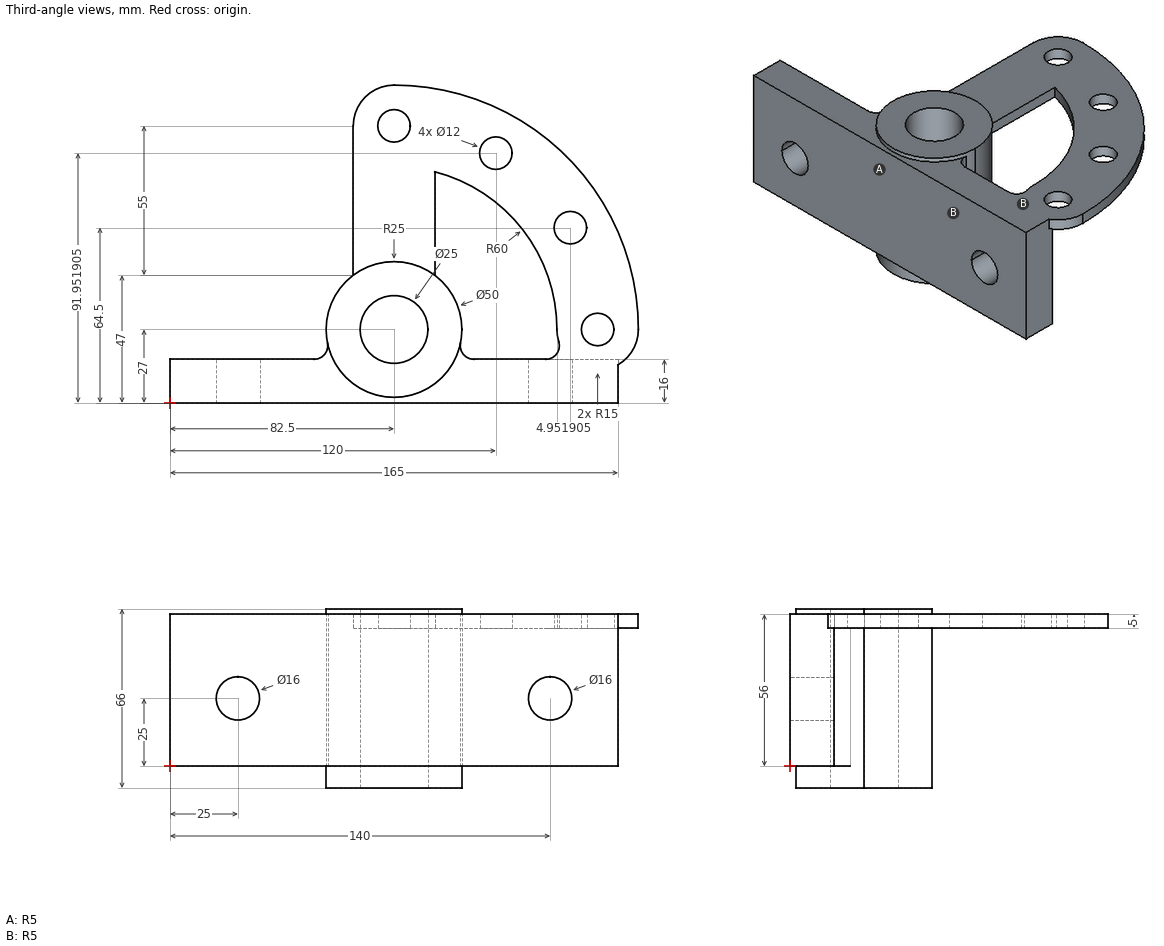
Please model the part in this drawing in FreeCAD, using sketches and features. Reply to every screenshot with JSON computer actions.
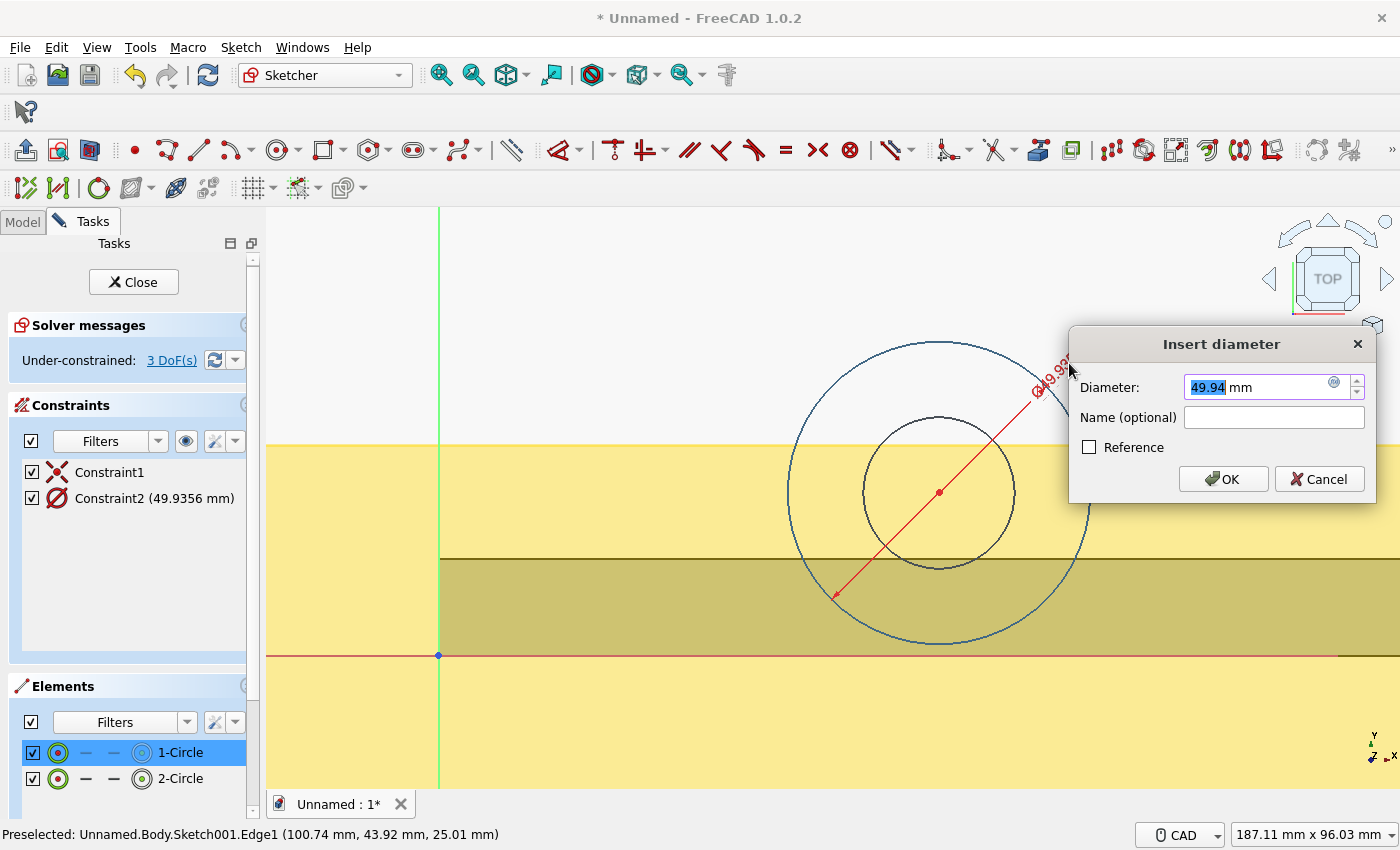
{"action": "type", "text": "50"}
{"action": "key", "text": "Return"}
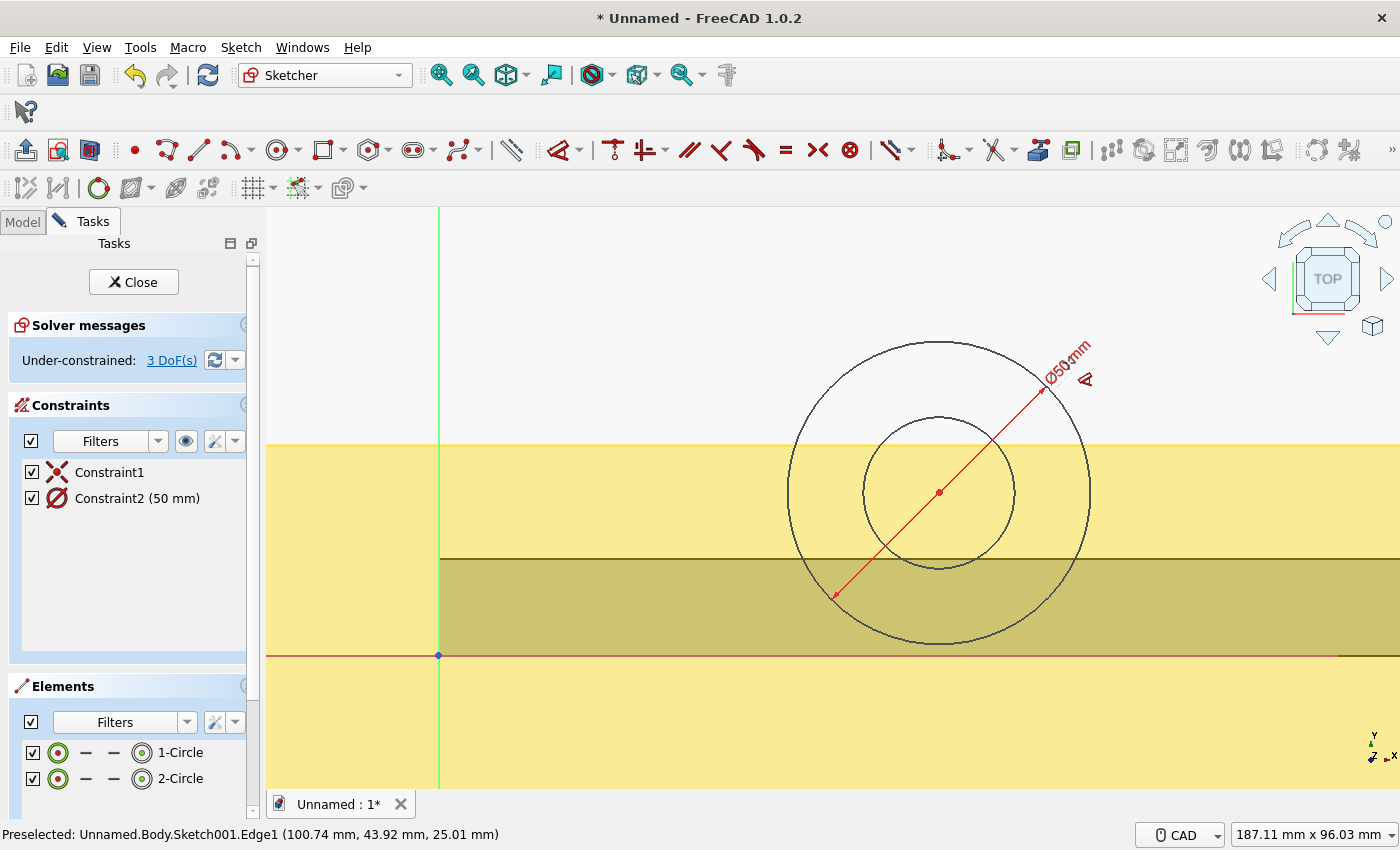
{"action": "left_click", "coordinate": [992, 439]}
{"action": "left_click", "coordinate": [1014, 416]}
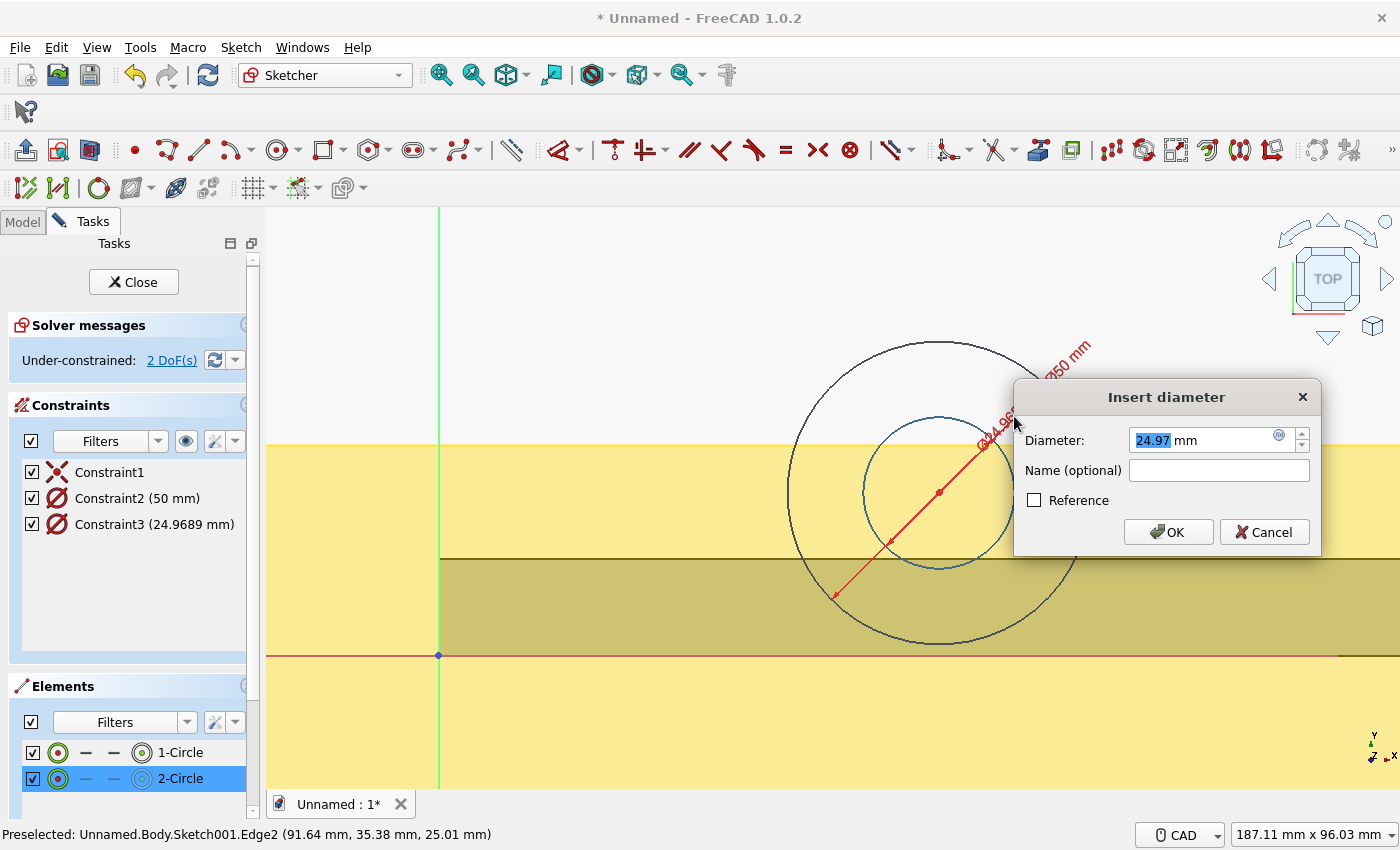
{"action": "type", "text": "25"}
{"action": "key", "text": "Return"}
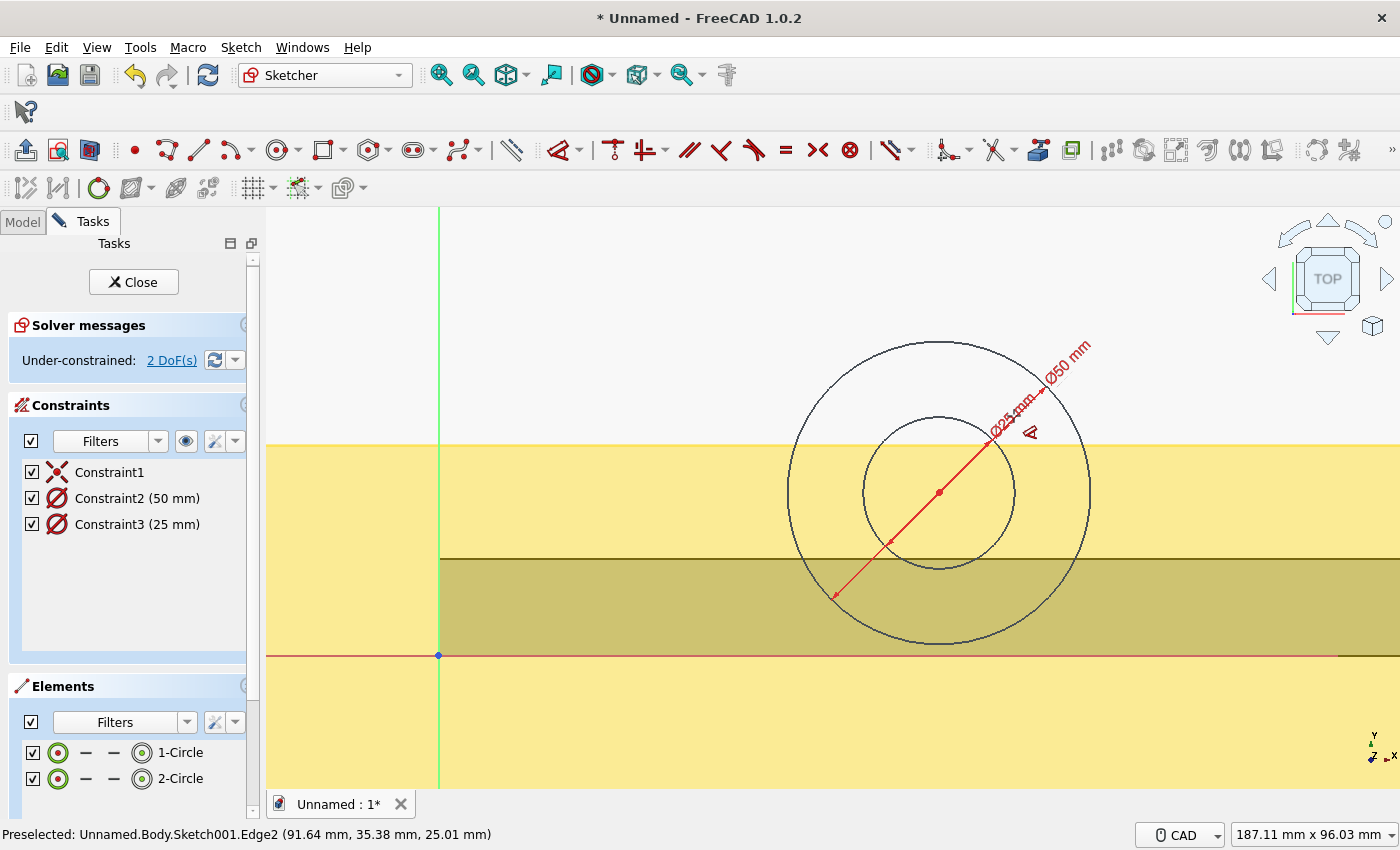
{"action": "left_click", "coordinate": [939, 493]}
{"action": "left_click", "coordinate": [405, 574]}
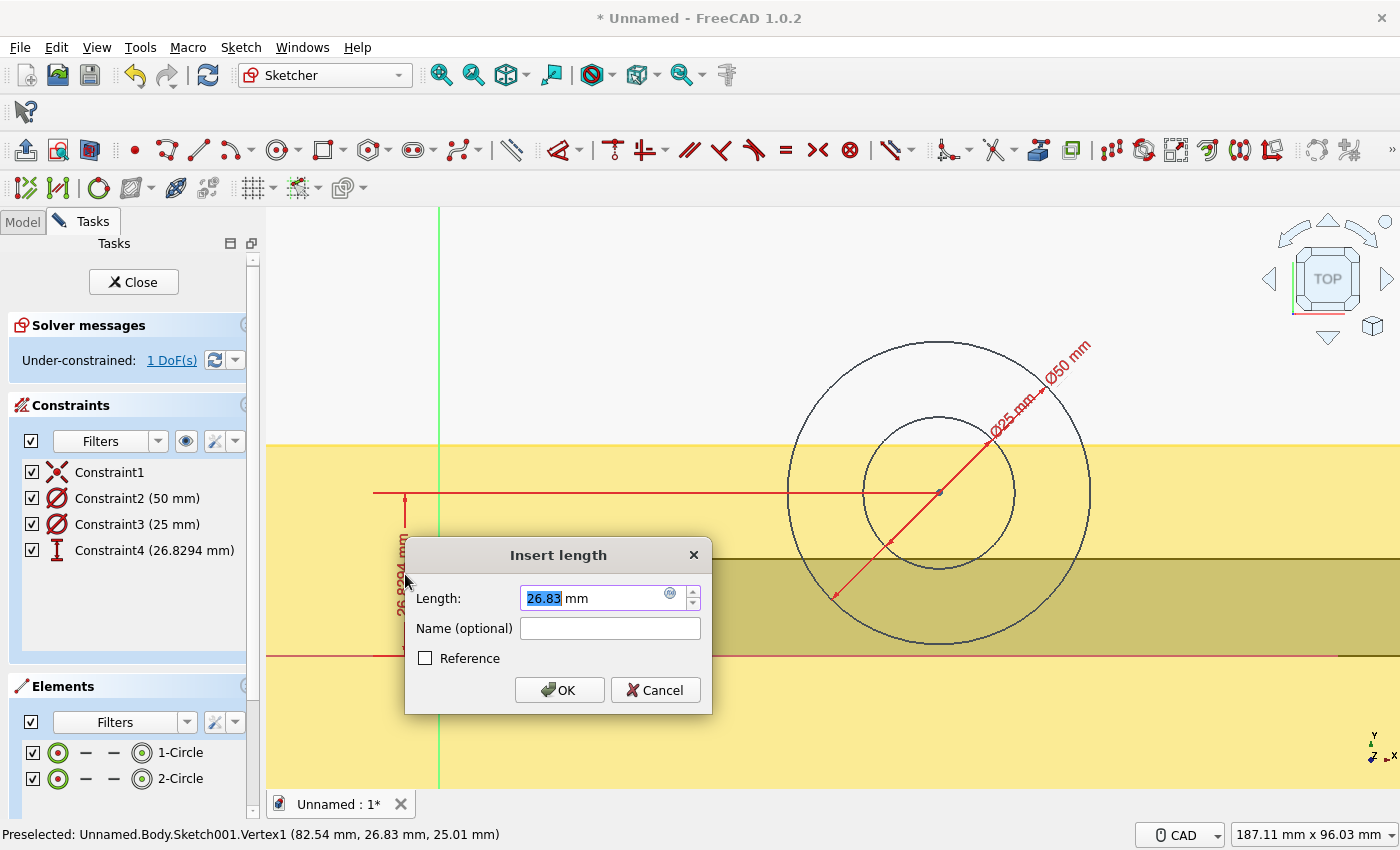
{"action": "type", "text": "27"}
{"action": "key", "text": "Return"}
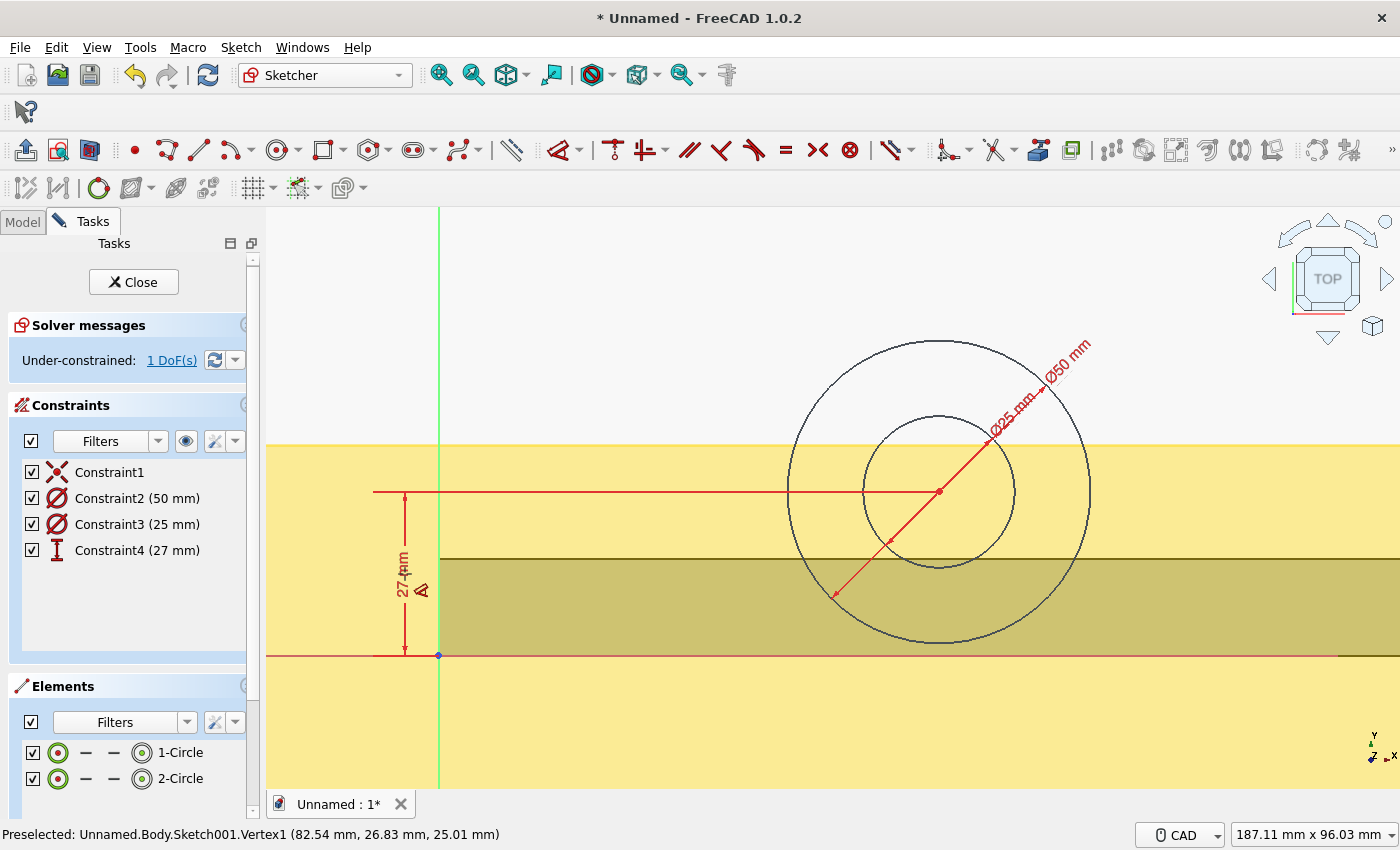
{"action": "left_click", "coordinate": [939, 492]}
{"action": "left_click", "coordinate": [689, 690]}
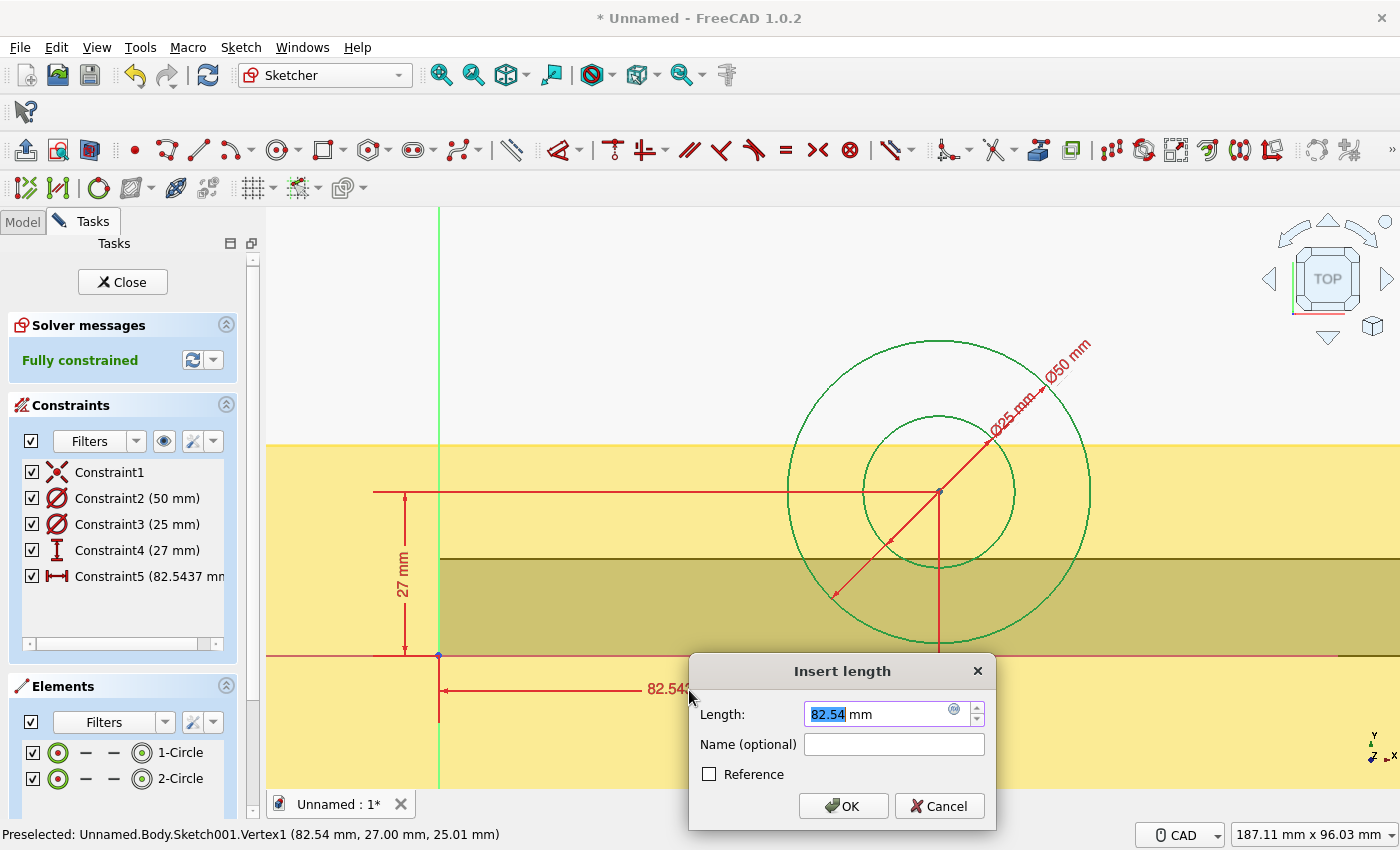
{"action": "type", "text": "82.5"}
{"action": "key", "text": "Return"}
{"action": "key", "text": "Escape"}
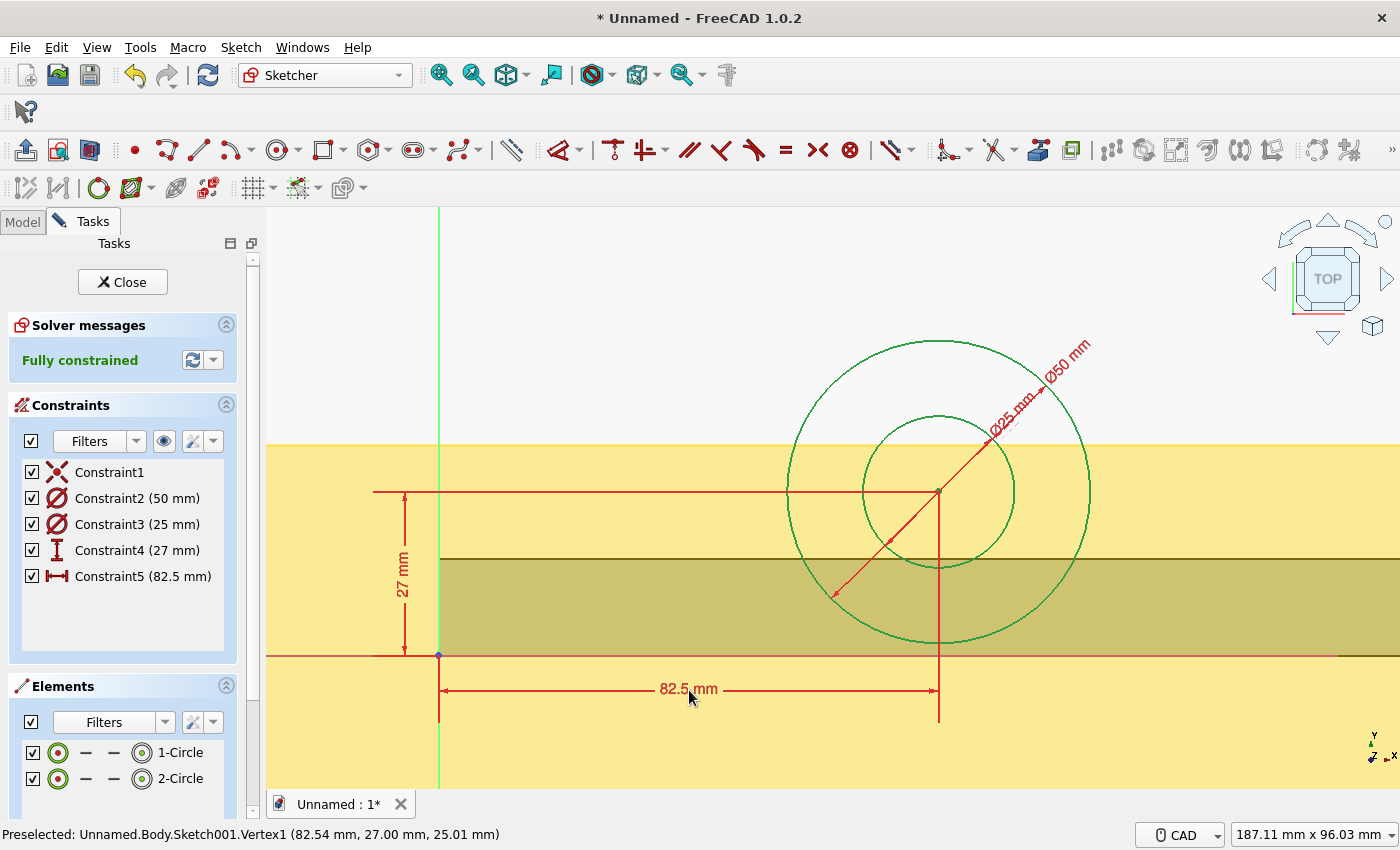
{"action": "left_click", "coordinate": [123, 282]}